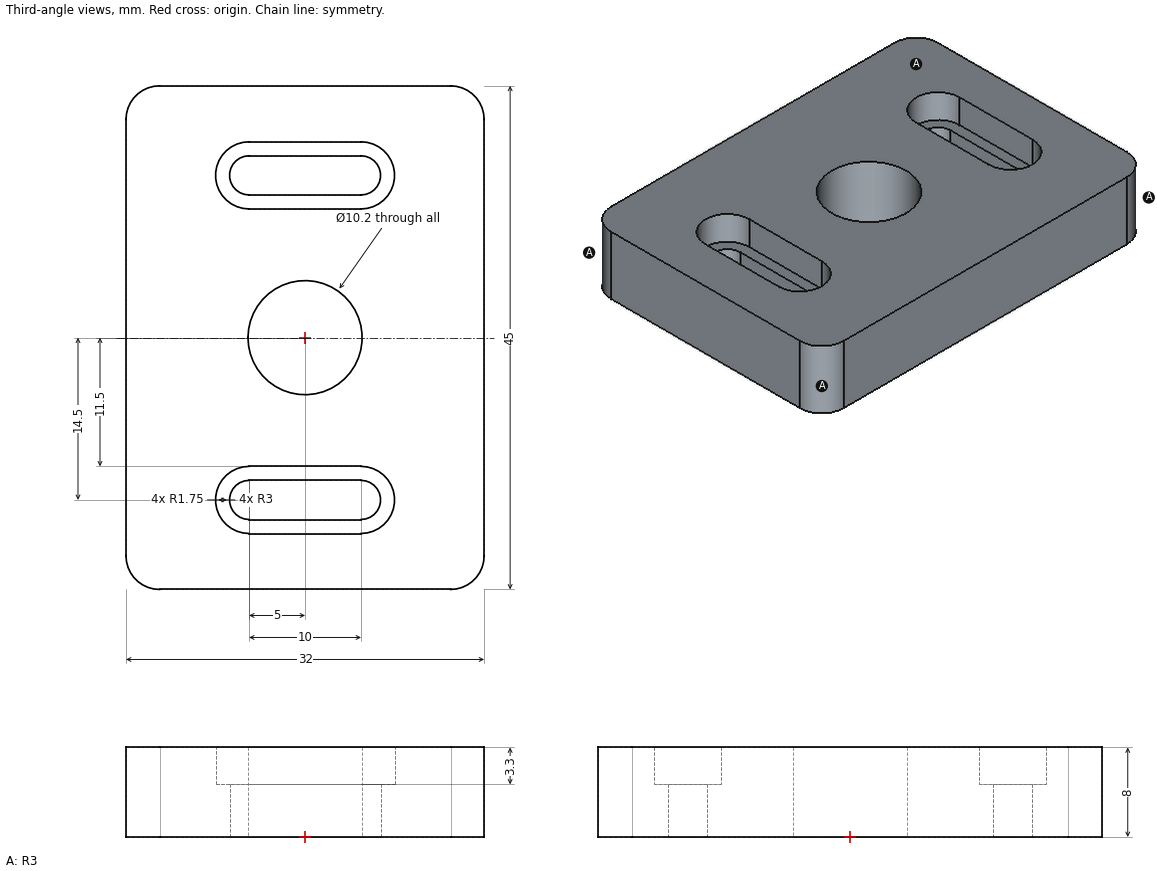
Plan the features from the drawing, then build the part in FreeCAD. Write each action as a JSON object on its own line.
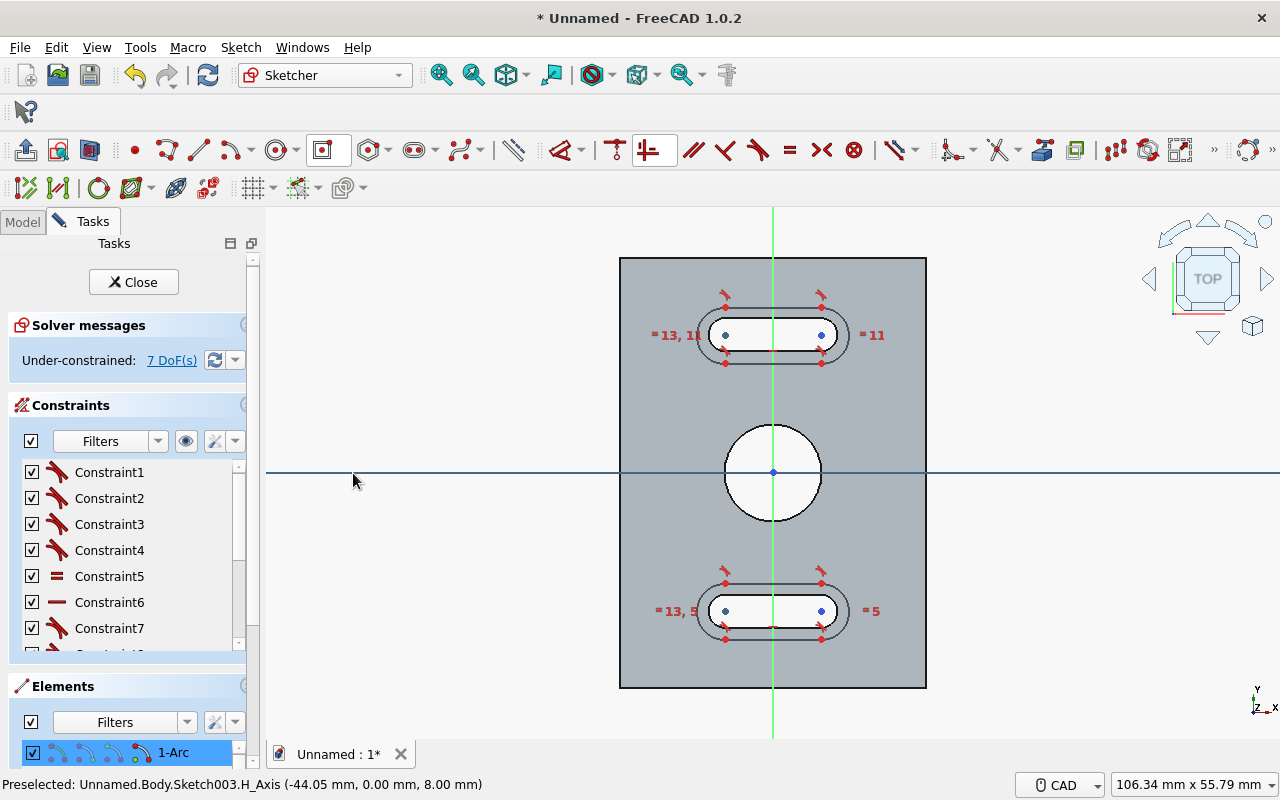
{"action": "left_click", "coordinate": [822, 150]}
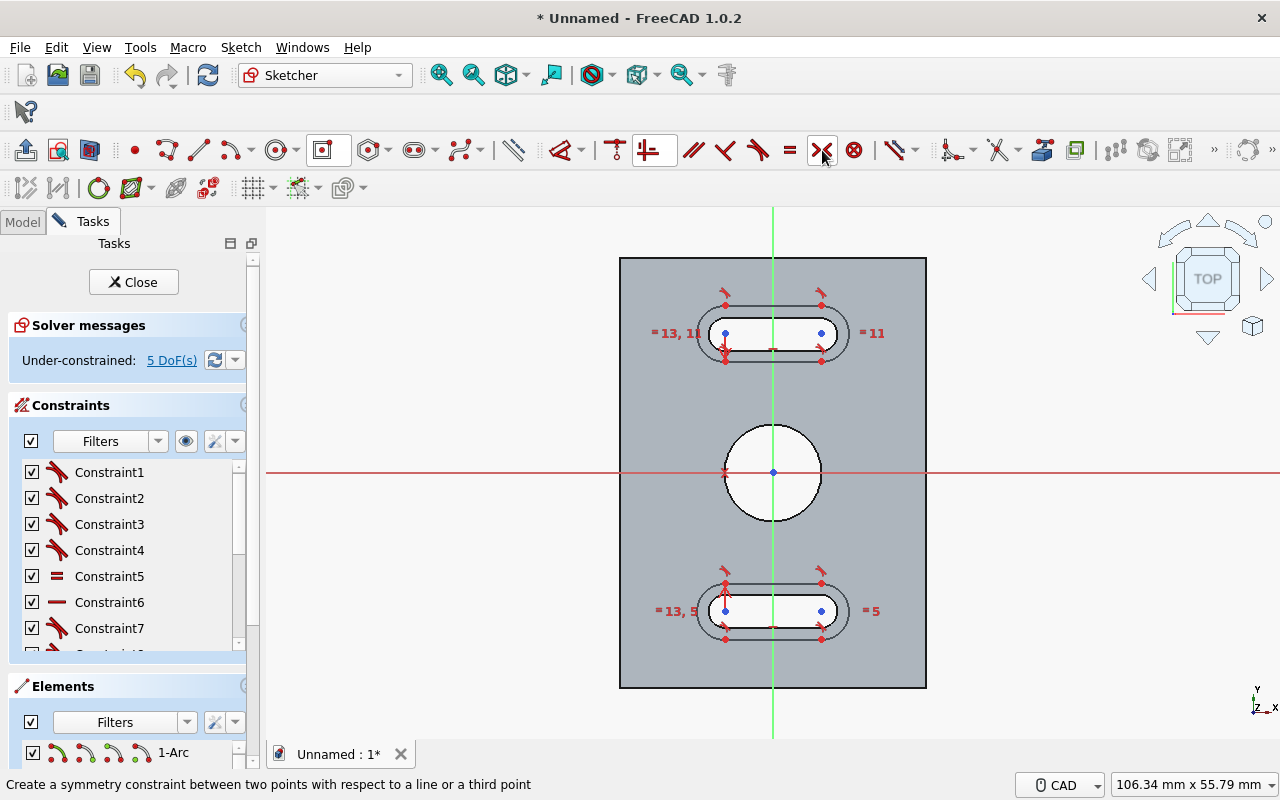
{"action": "left_click", "coordinate": [560, 150]}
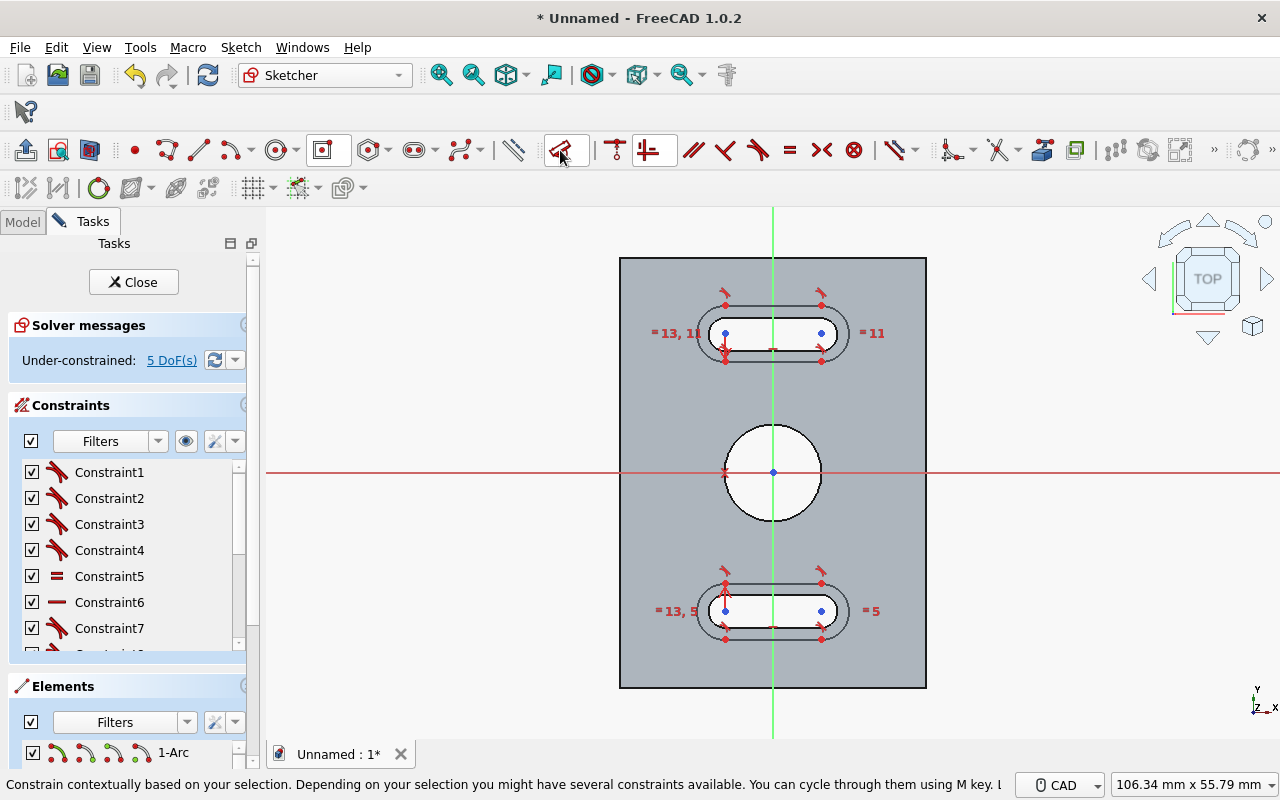
{"action": "scroll", "coordinate": [702, 596], "scroll_direction": "up", "scroll_amount": 2}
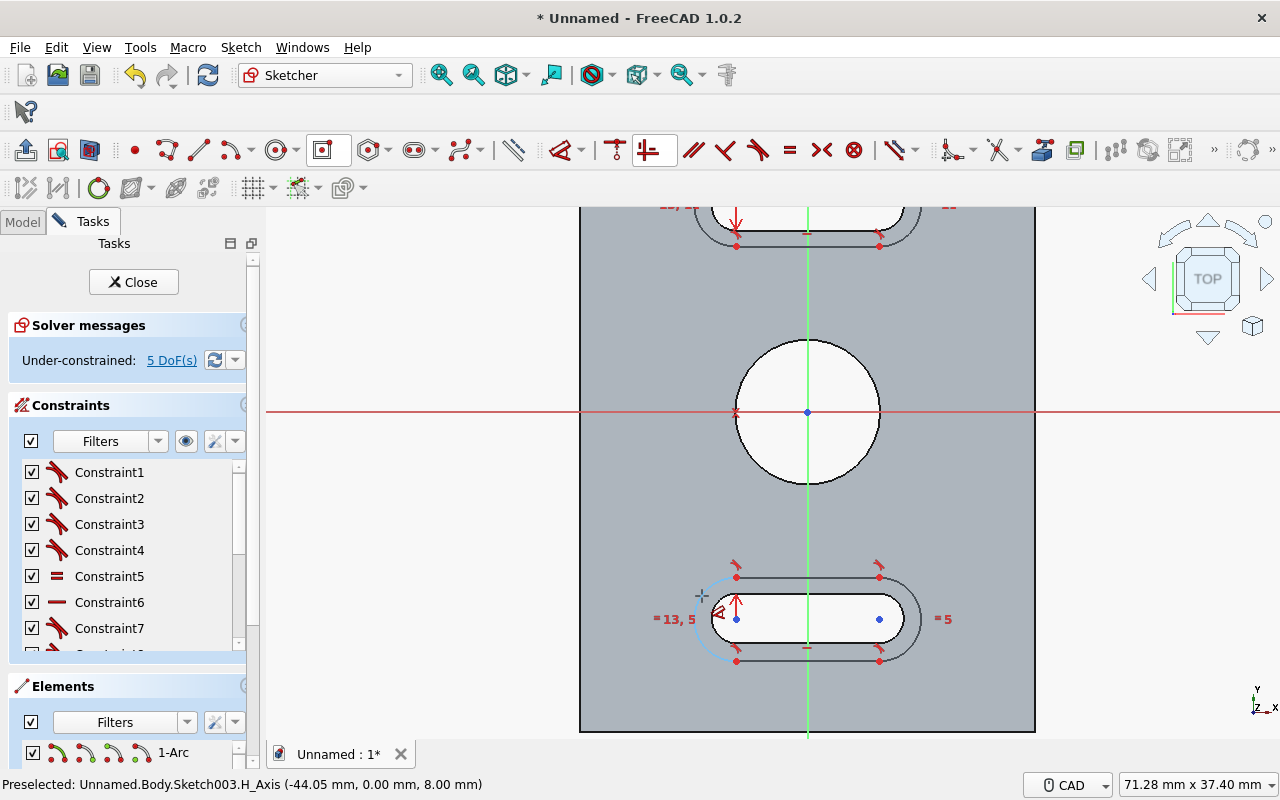
{"action": "left_click", "coordinate": [702, 595]}
{"action": "left_click", "coordinate": [676, 576]}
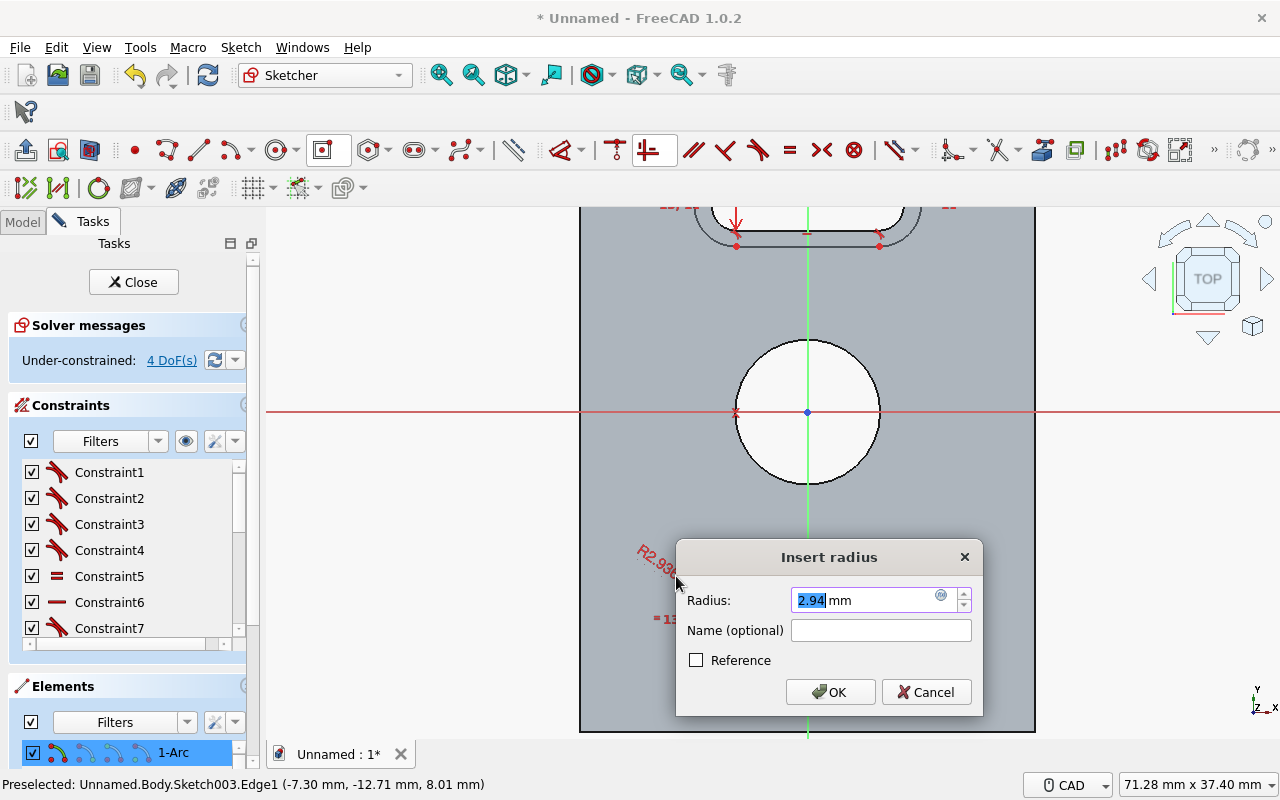
{"action": "type", "text": "3"}
{"action": "key", "text": "Return"}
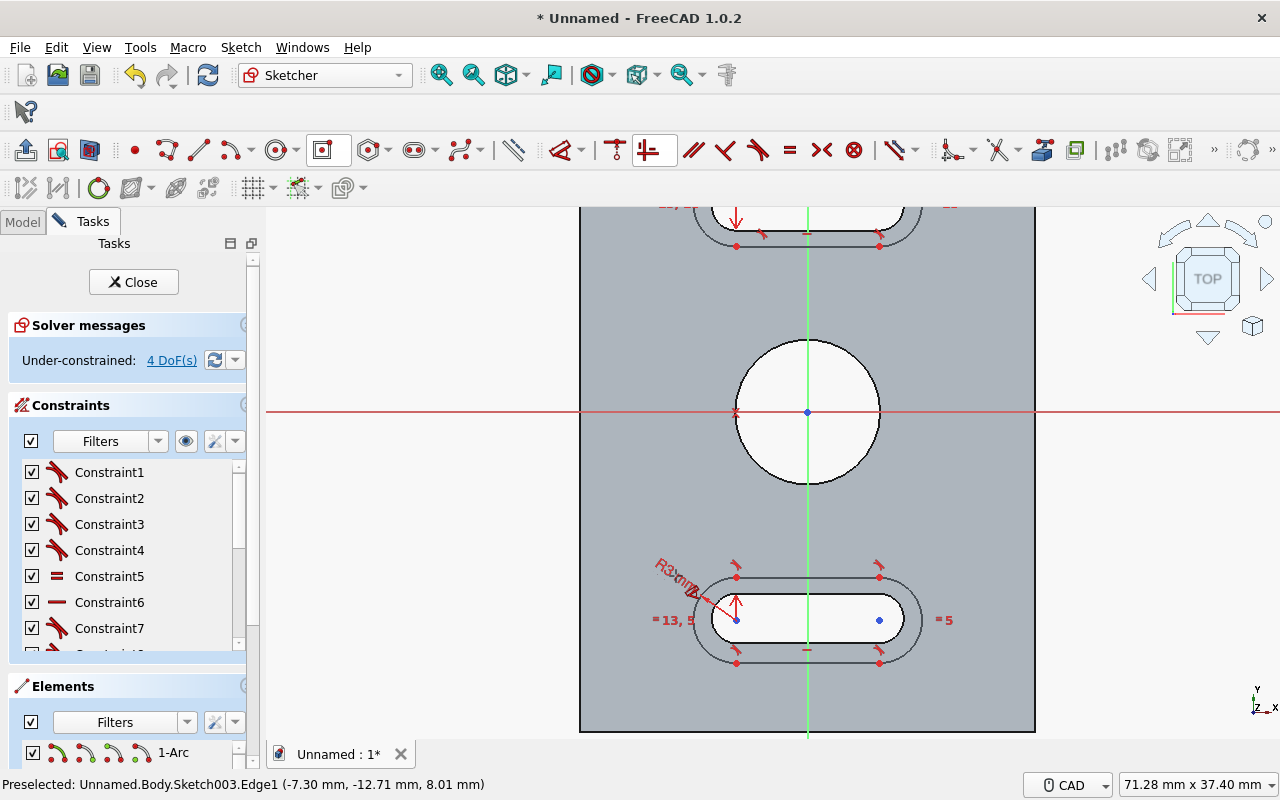
{"action": "left_click", "coordinate": [779, 578]}
{"action": "left_click", "coordinate": [775, 612]}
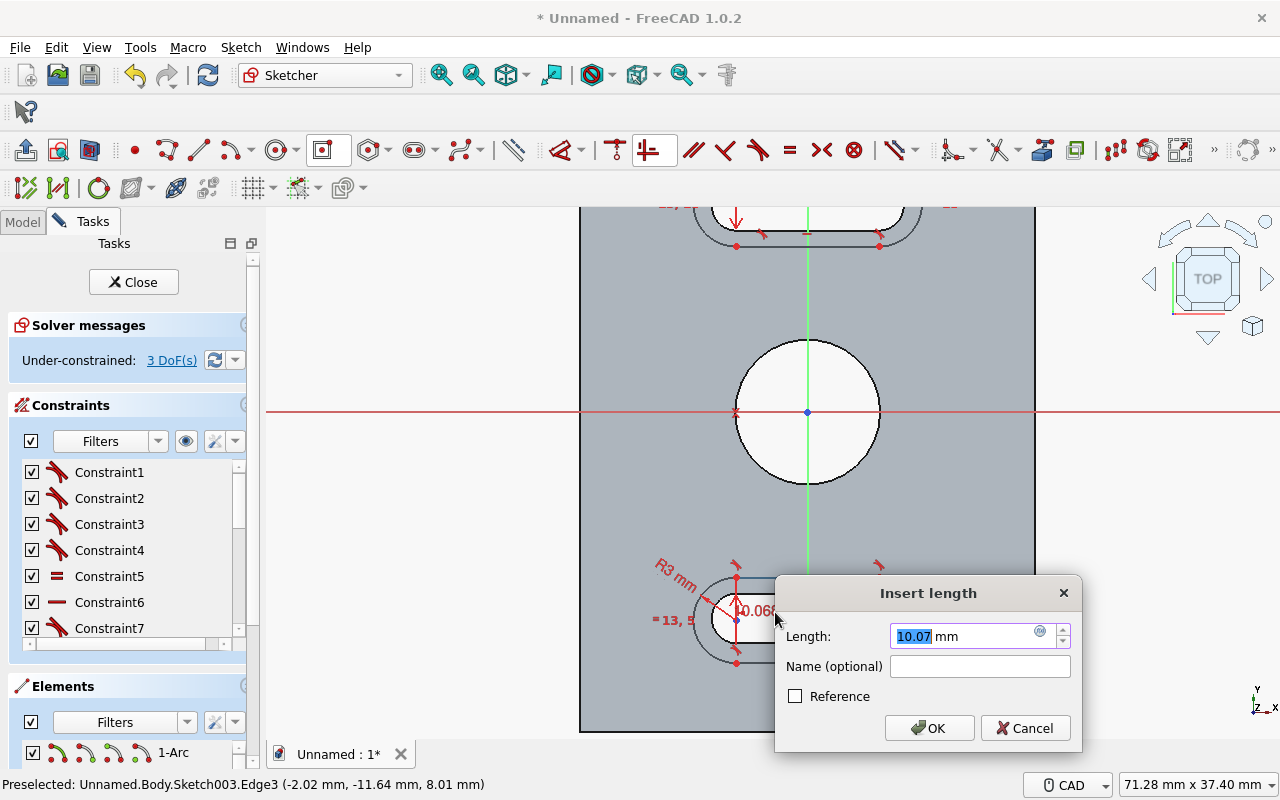
{"action": "type", "text": "10"}
{"action": "key", "text": "Return"}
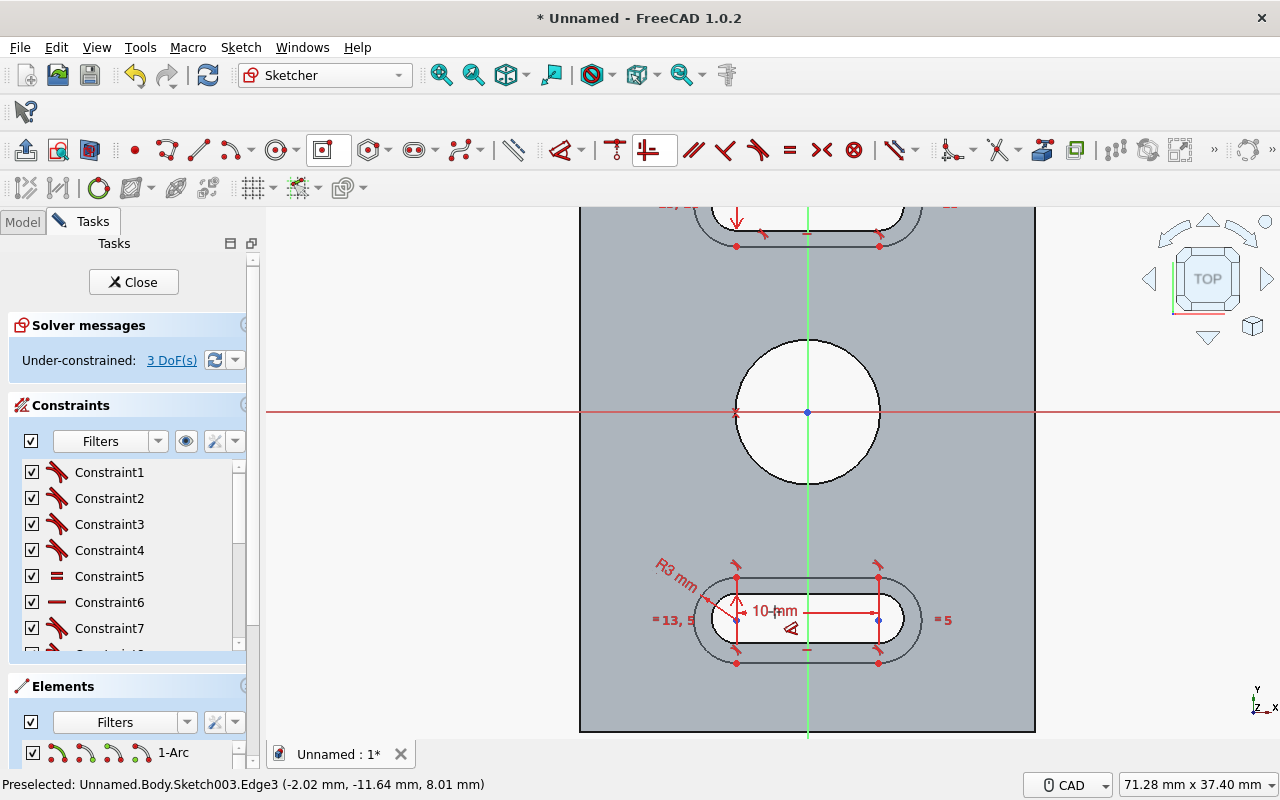
{"action": "scroll", "coordinate": [495, 597], "scroll_direction": "down", "scroll_amount": 2}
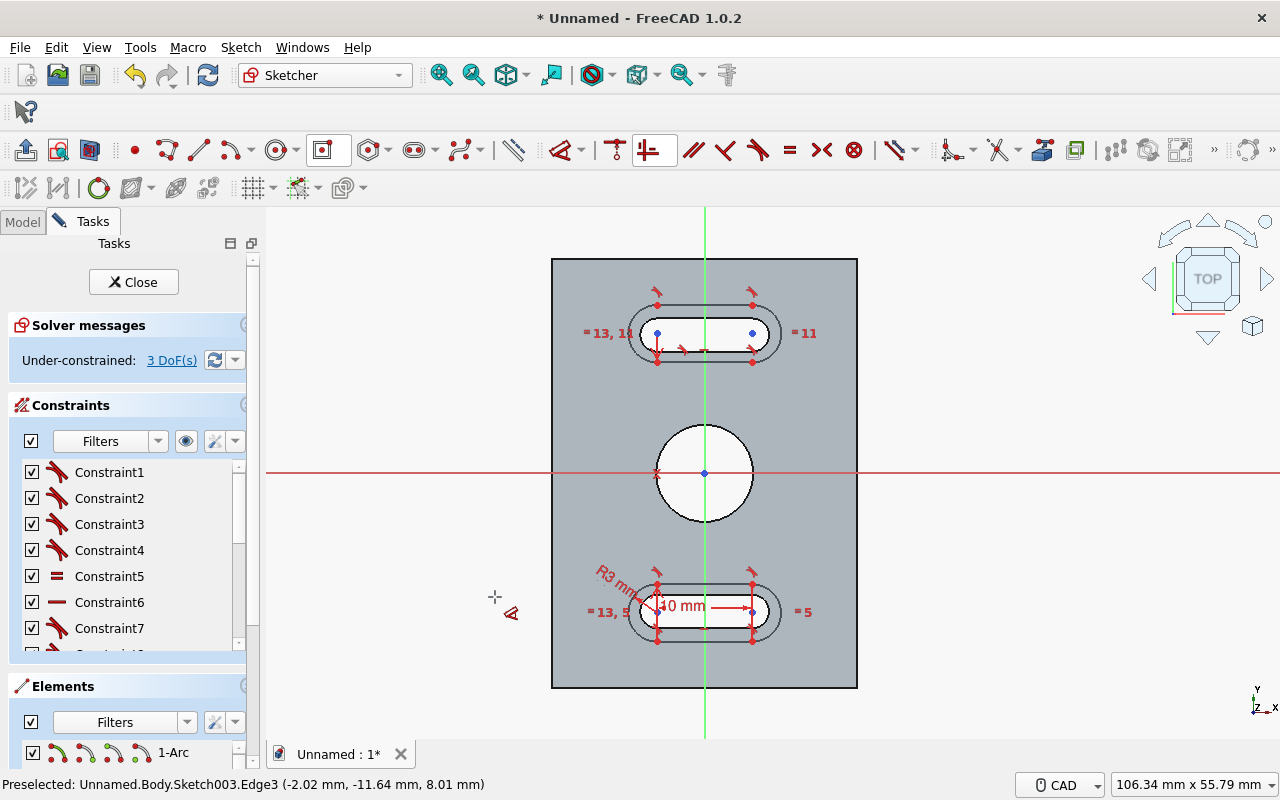
{"action": "left_click", "coordinate": [686, 305]}
{"action": "left_click", "coordinate": [683, 271]}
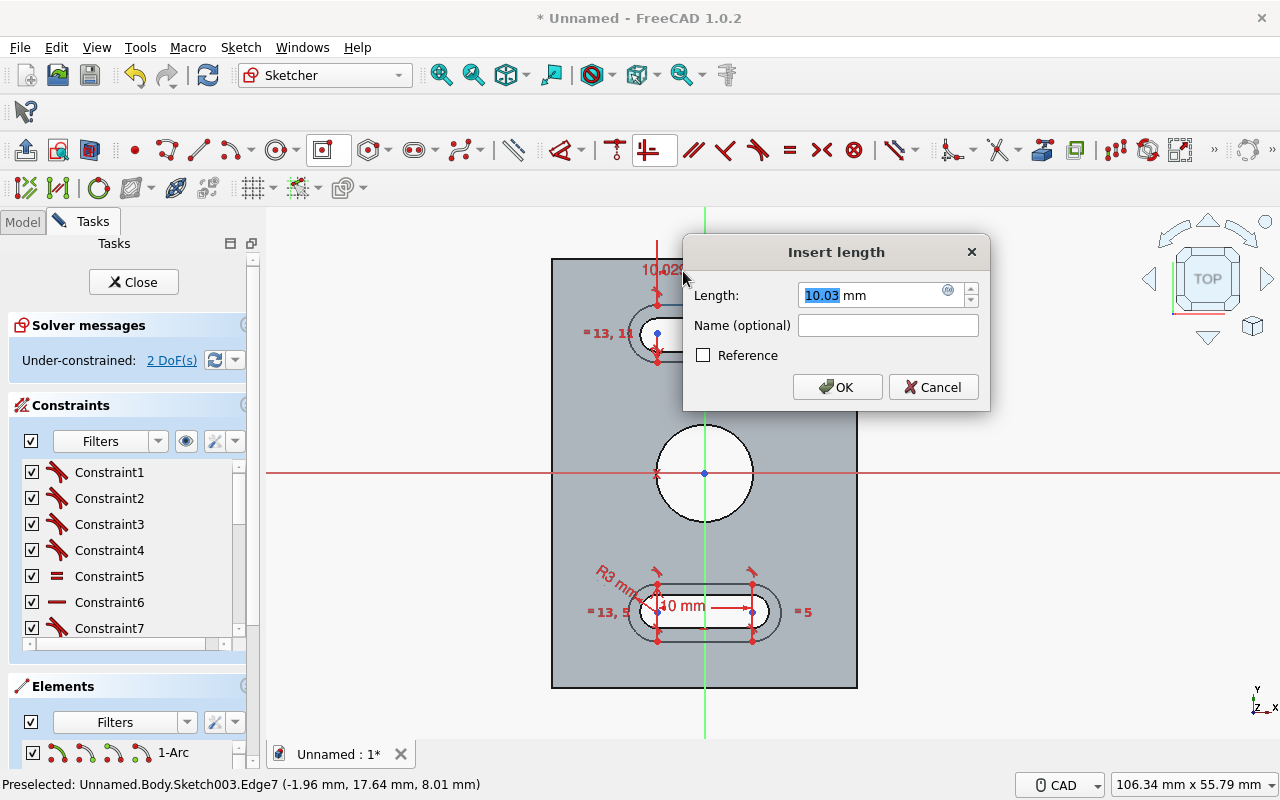
{"action": "type", "text": "10"}
{"action": "key", "text": "Return"}